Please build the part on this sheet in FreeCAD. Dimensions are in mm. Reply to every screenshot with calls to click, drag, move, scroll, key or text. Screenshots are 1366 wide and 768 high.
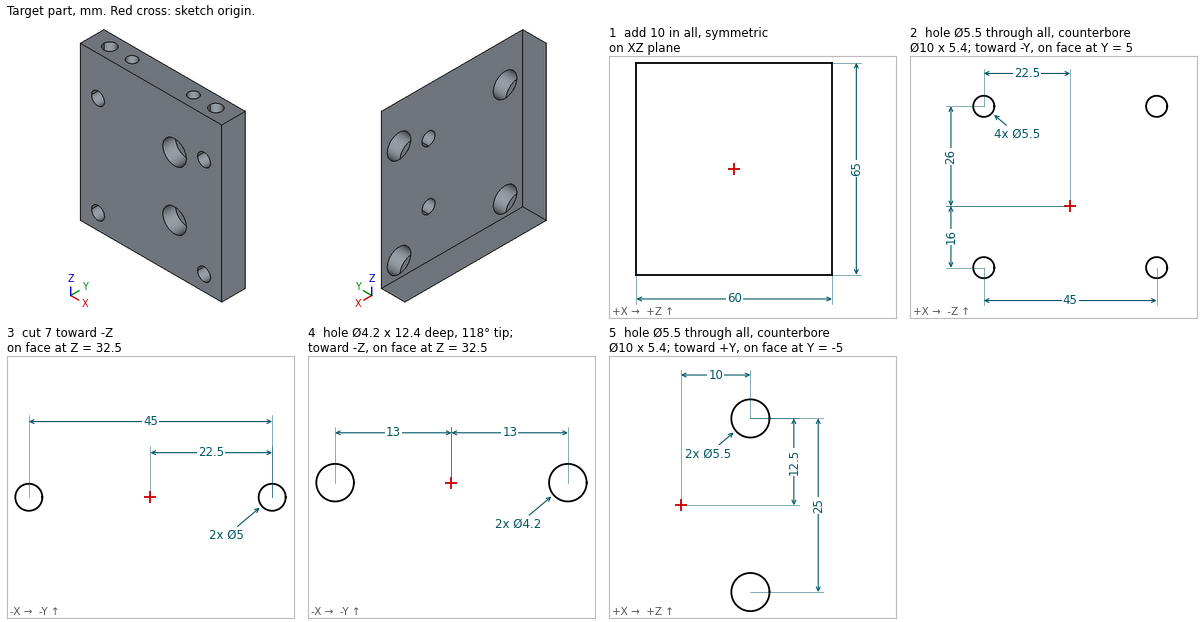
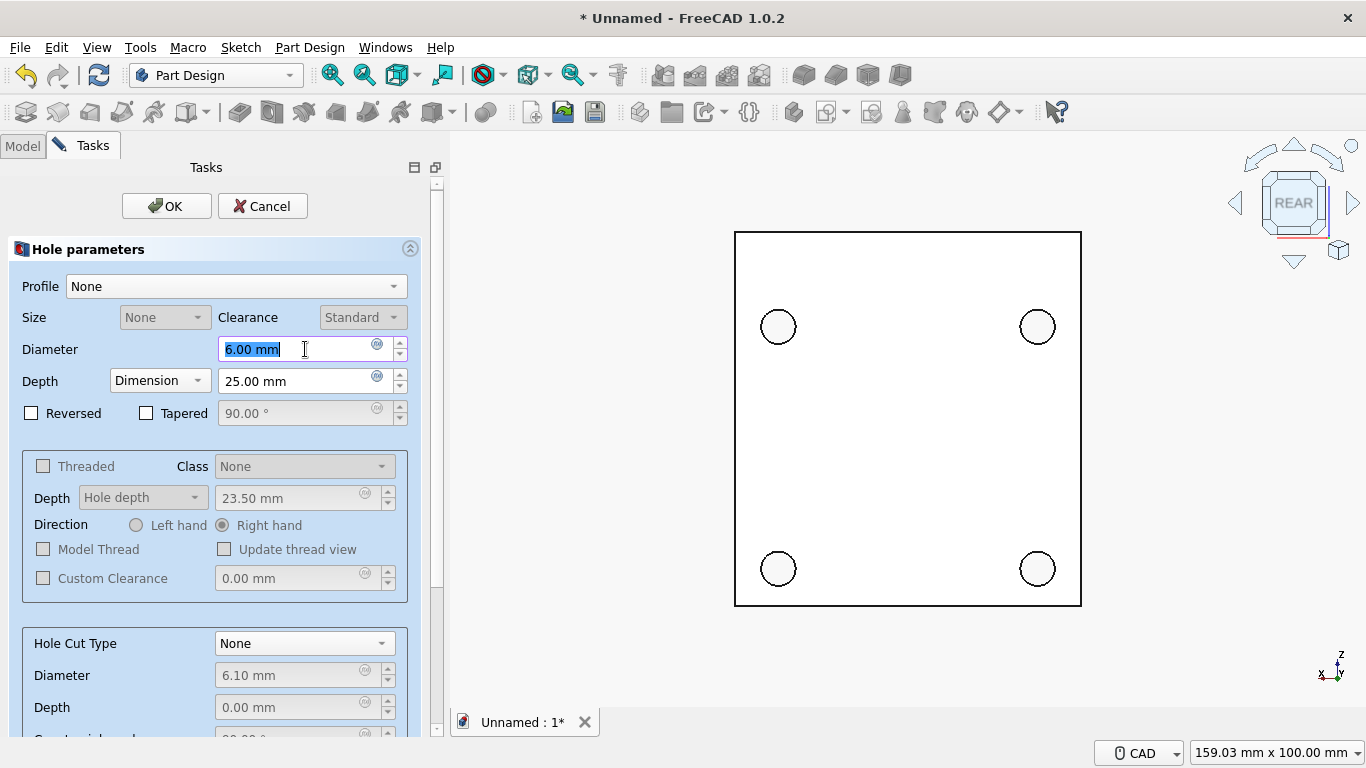
text(5.5)
key(Tab)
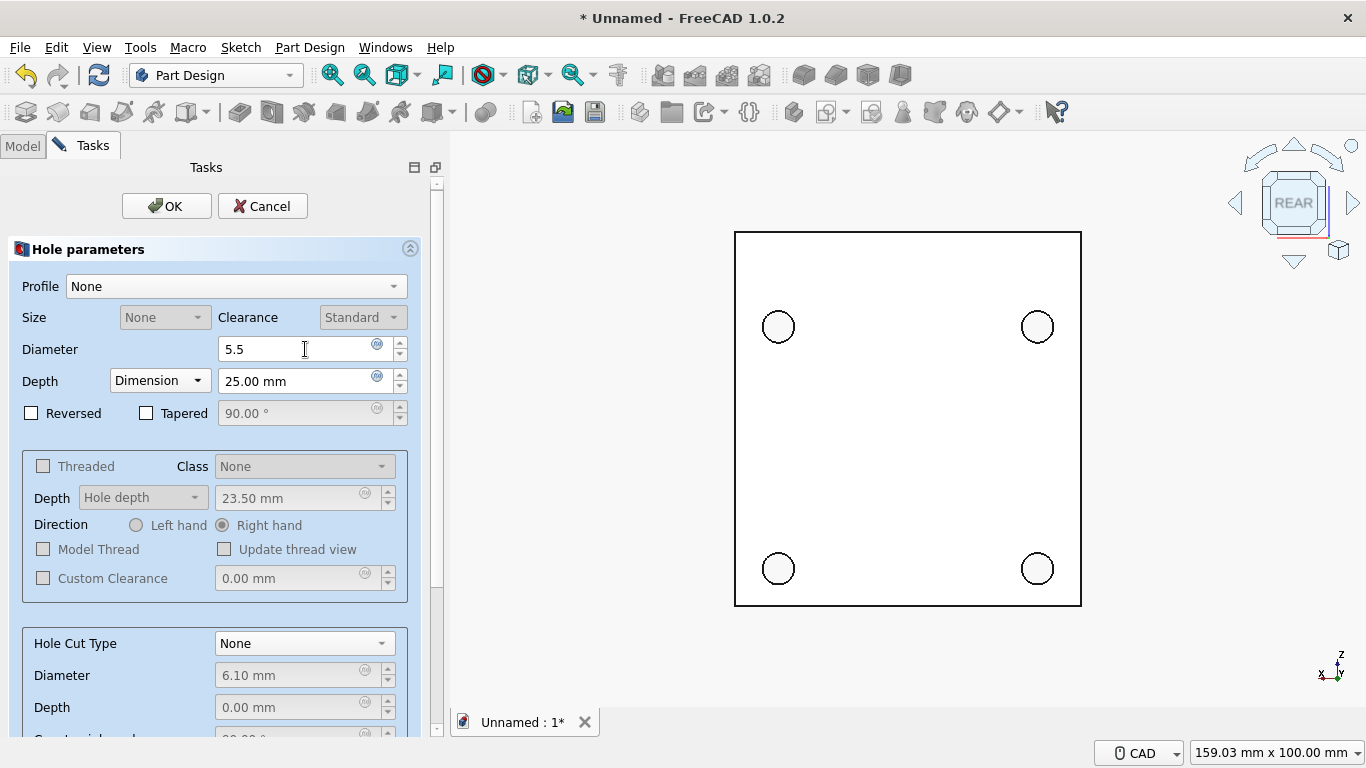
click(161, 380)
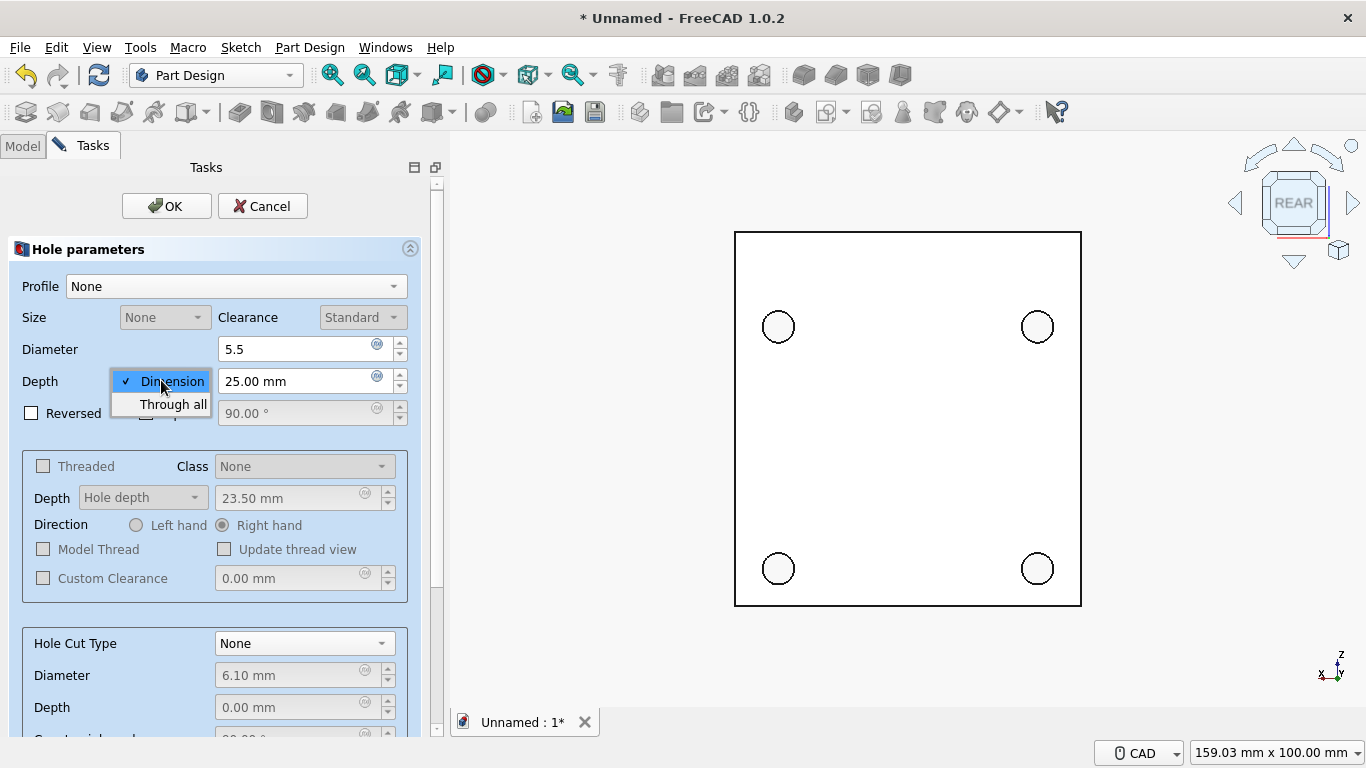
click(160, 404)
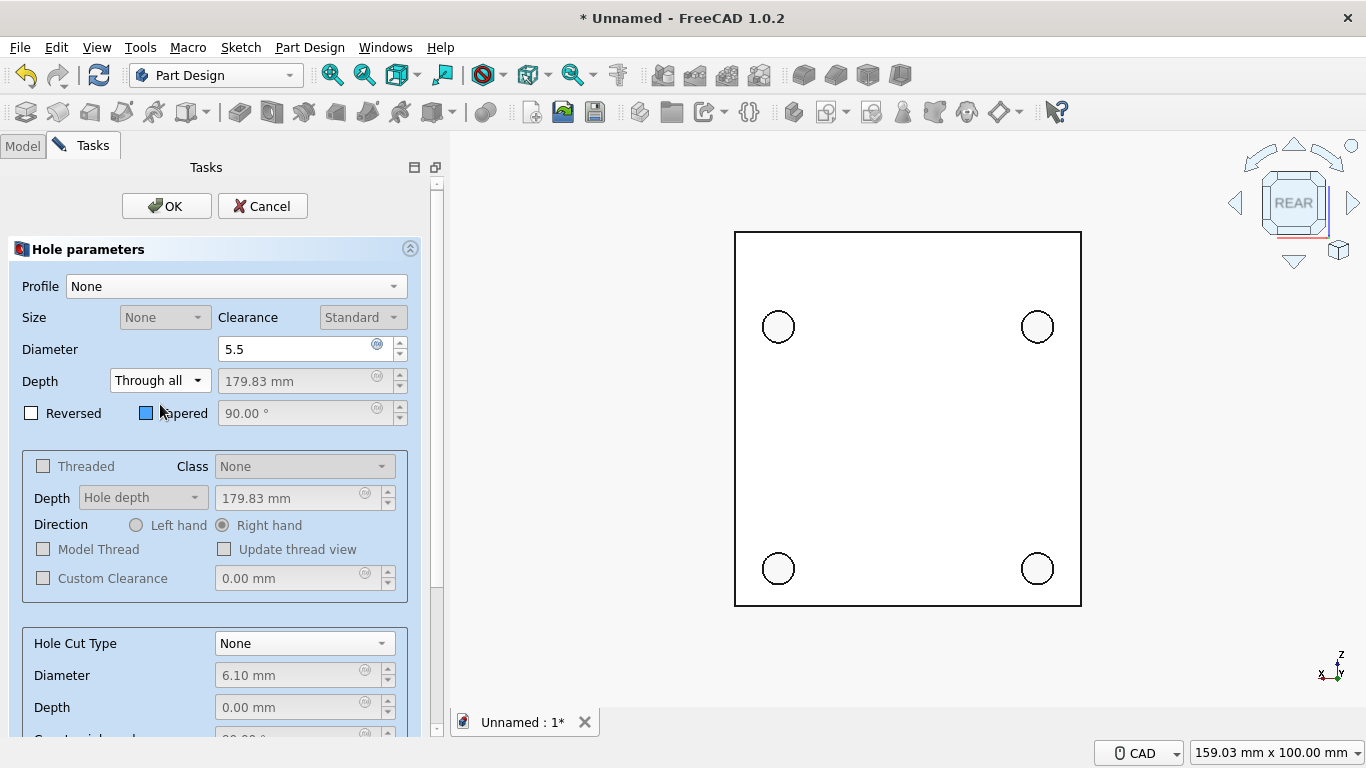
click(306, 644)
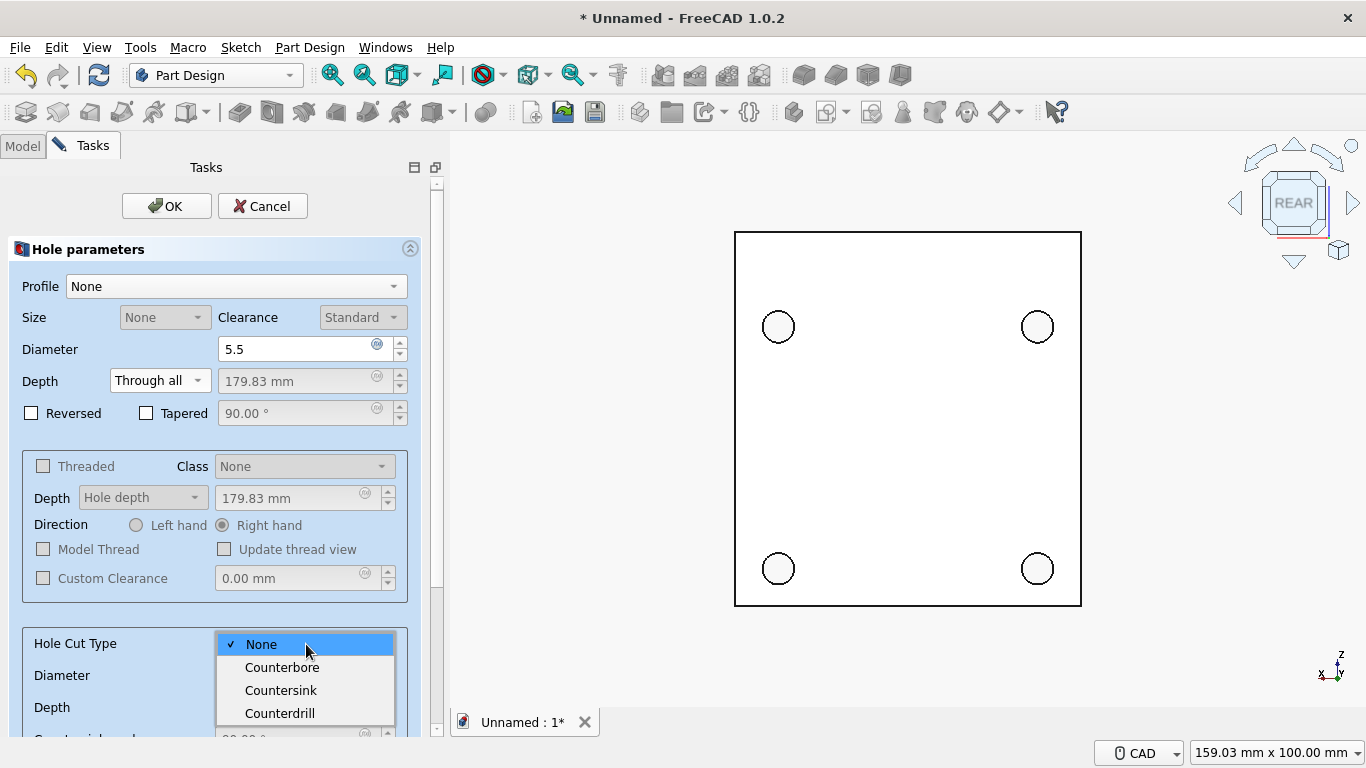
click(304, 668)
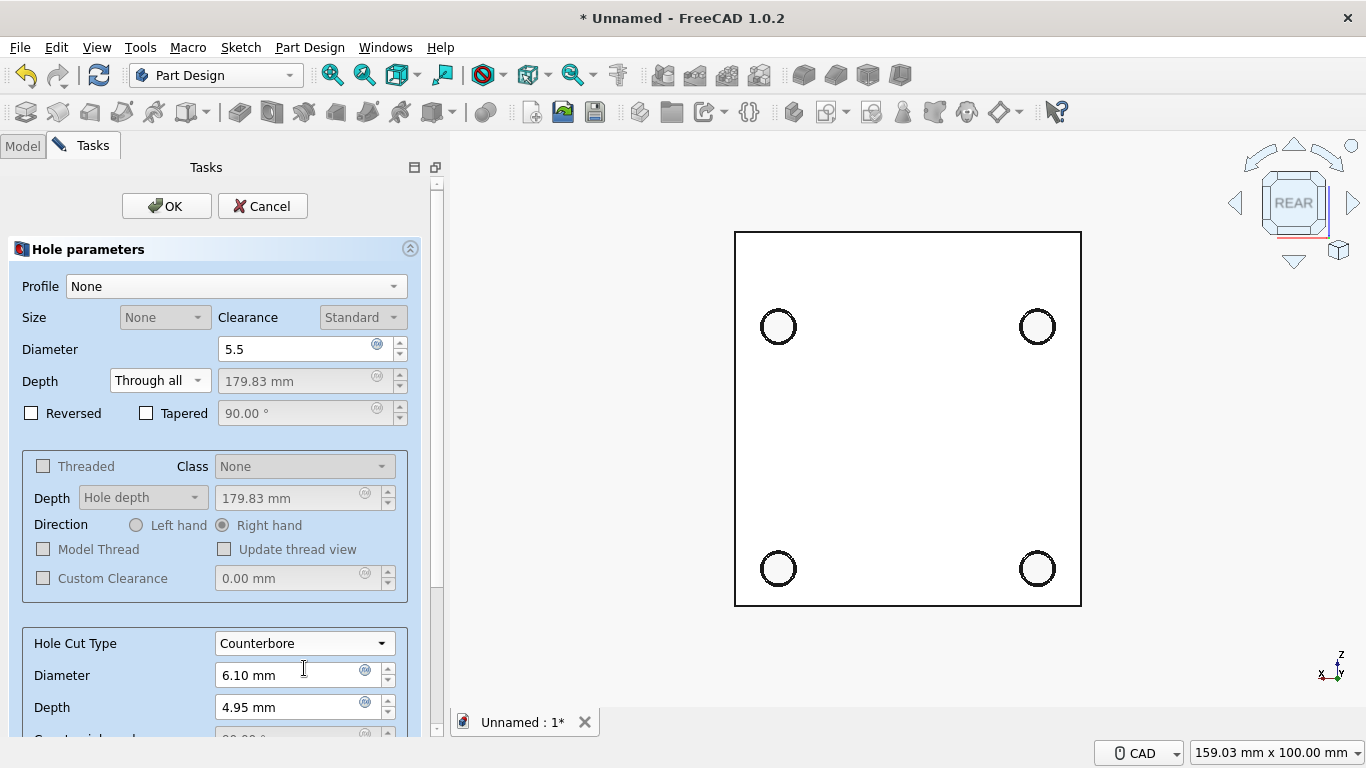
triple_click(298, 675)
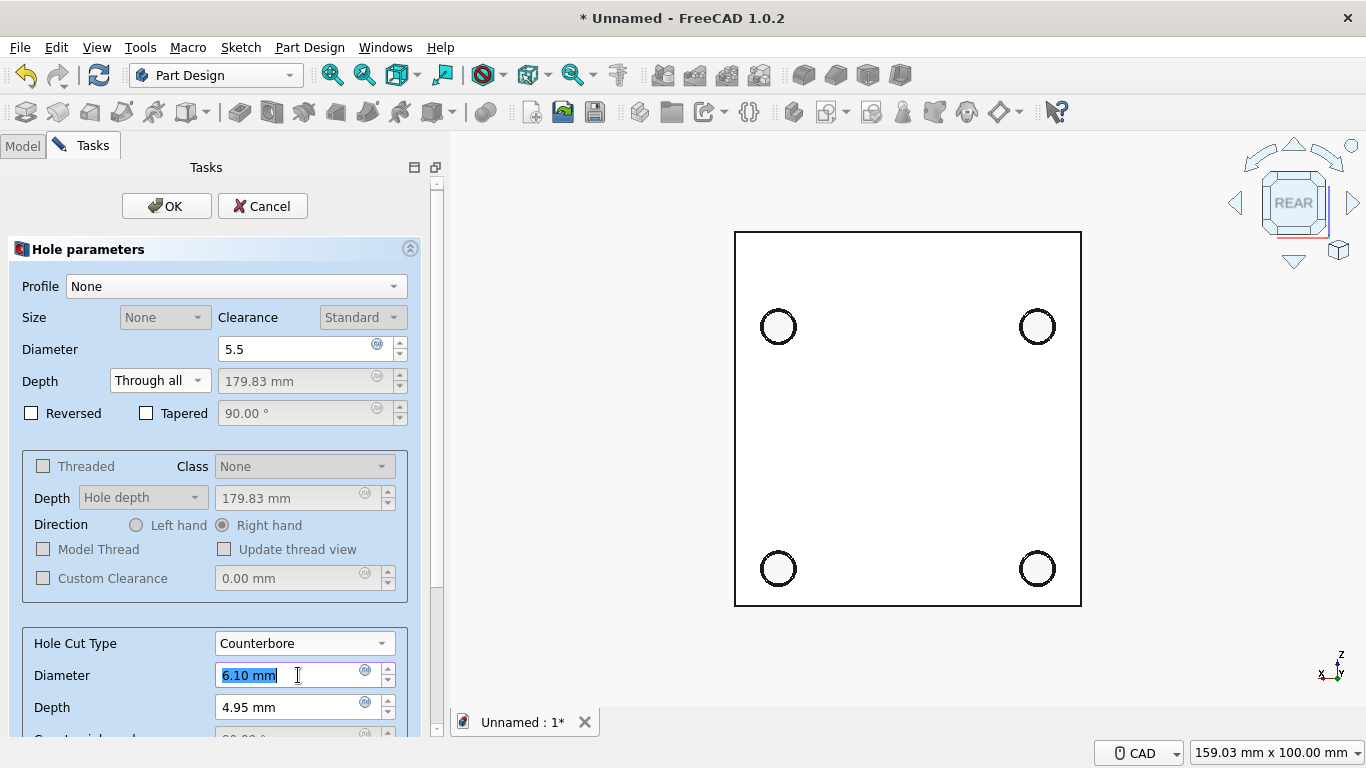
text(10)
key(Tab)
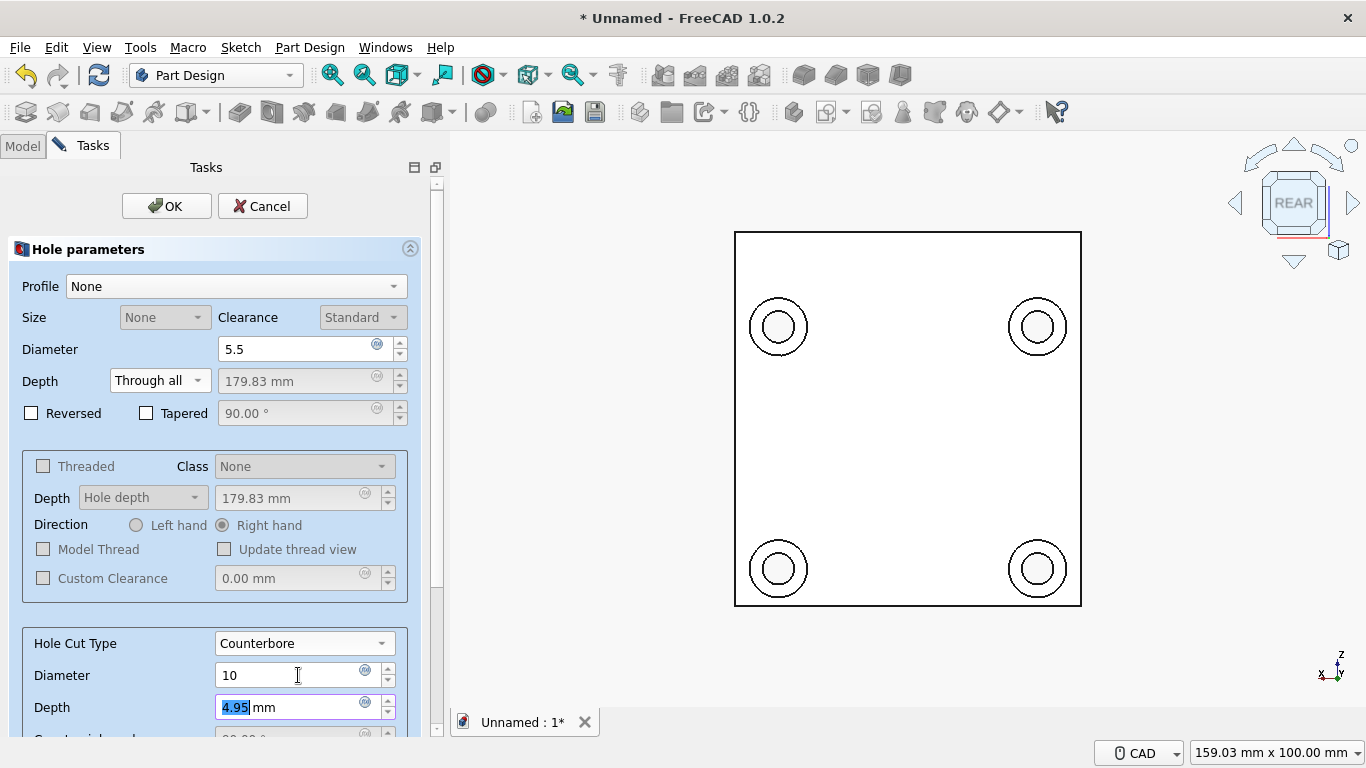
text(5.4)
key(Tab)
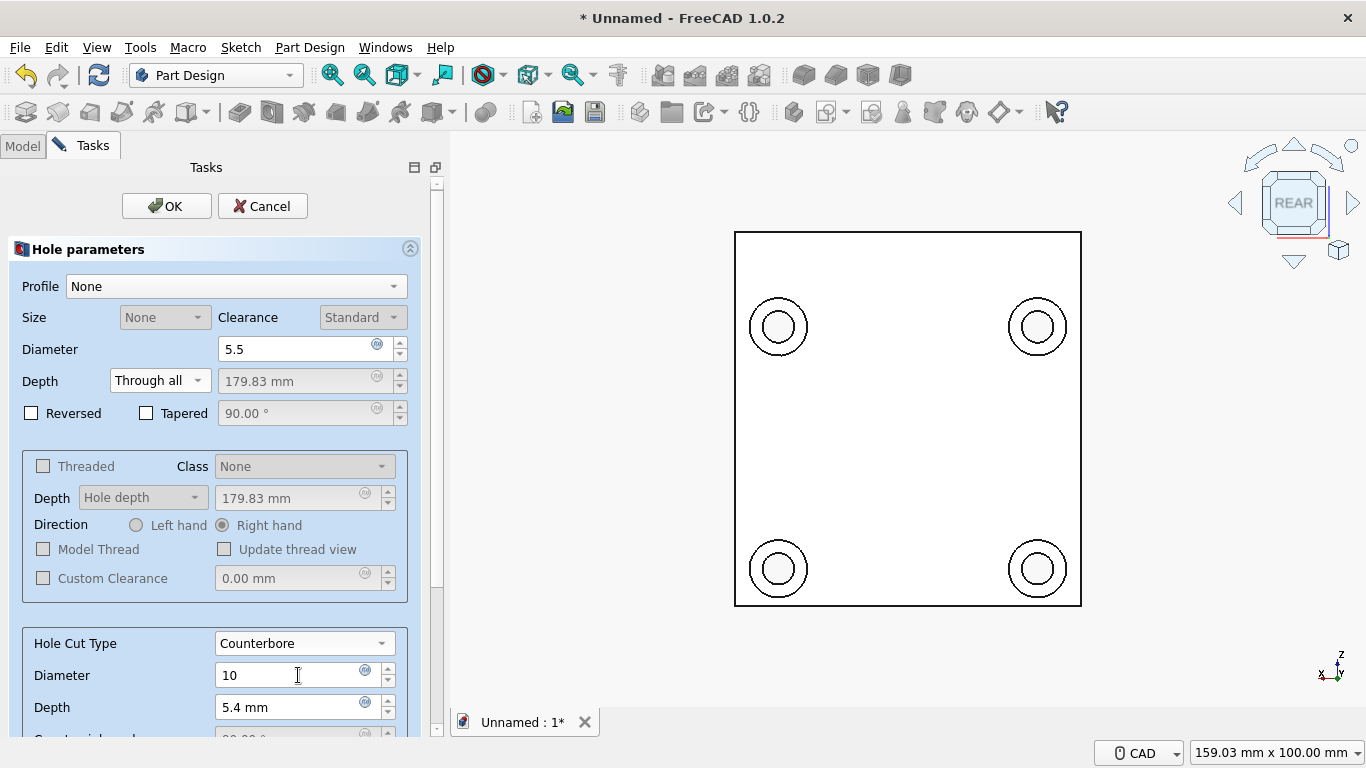
click(167, 206)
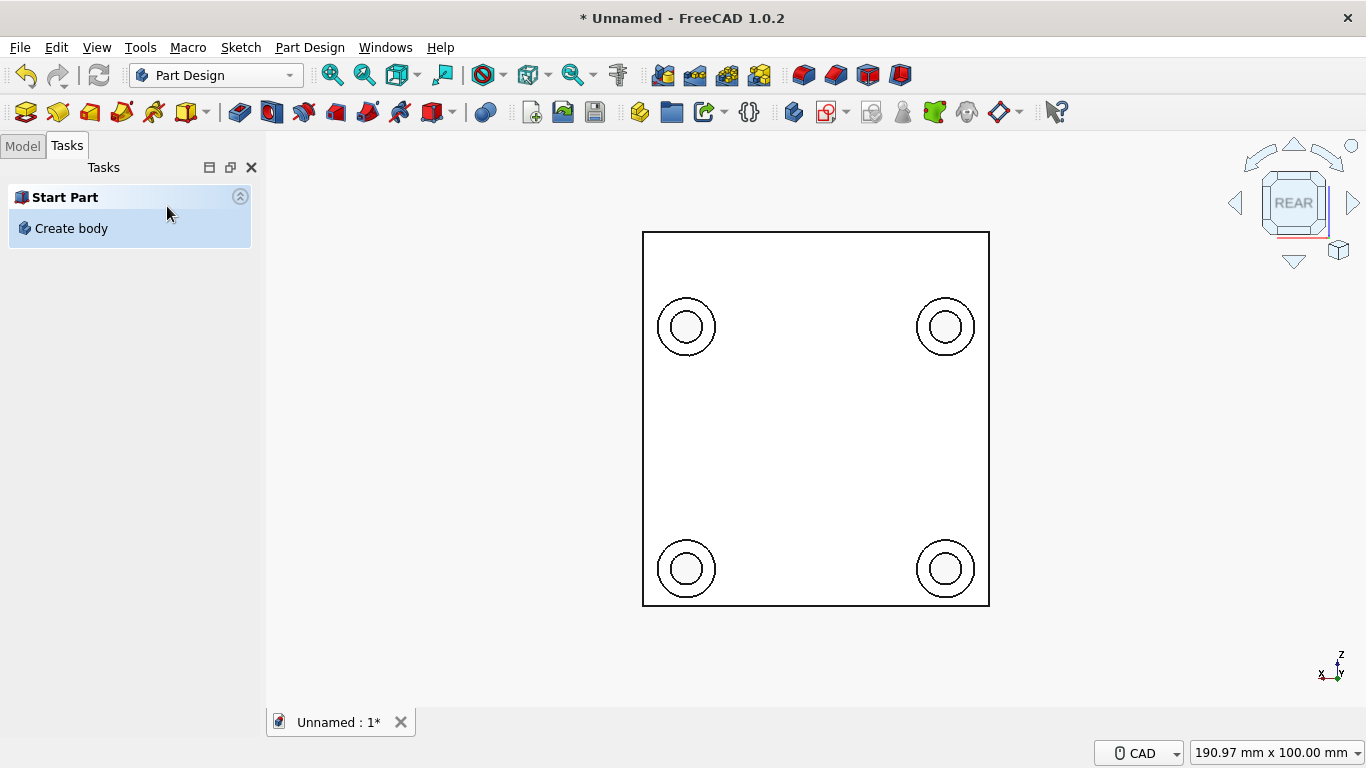
key(0)